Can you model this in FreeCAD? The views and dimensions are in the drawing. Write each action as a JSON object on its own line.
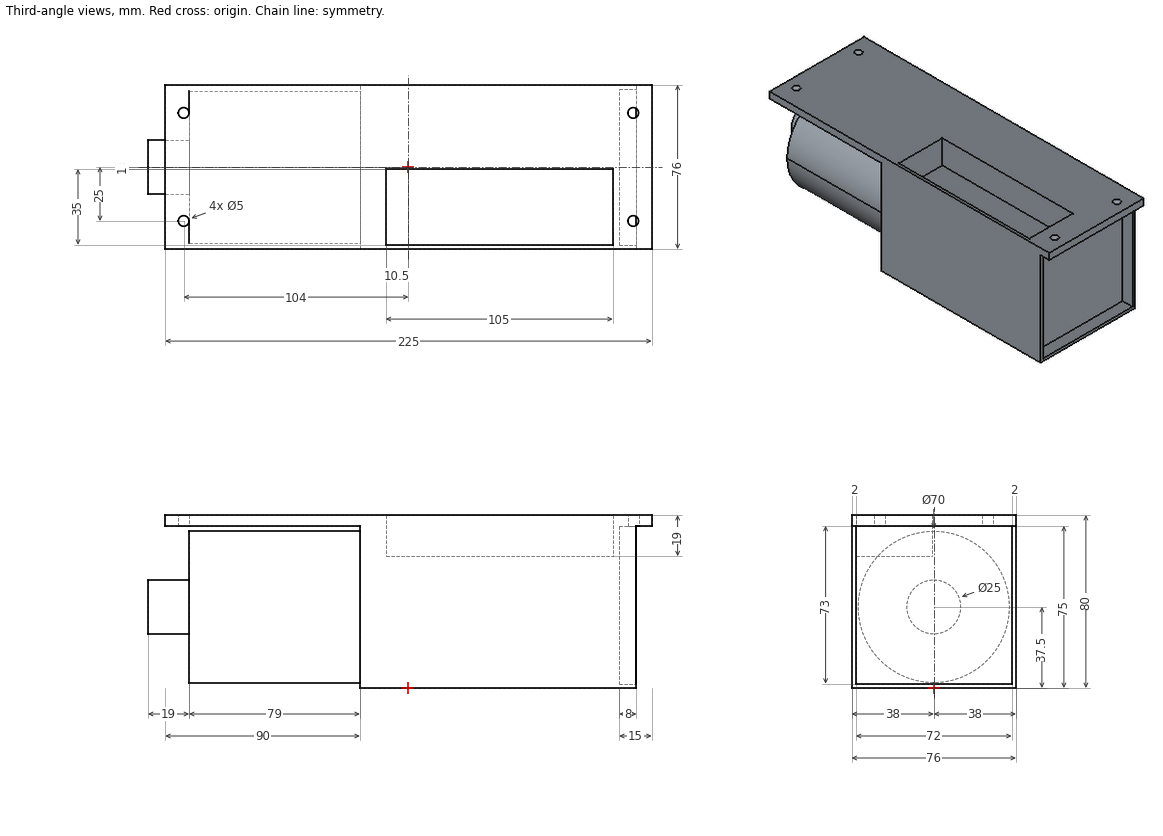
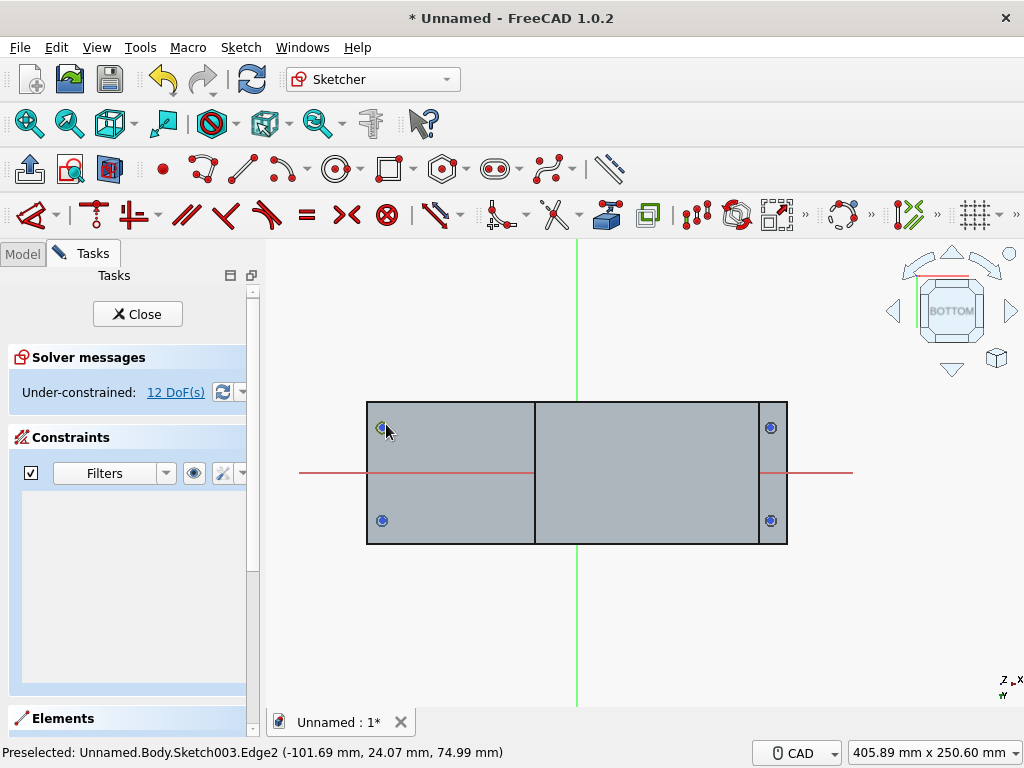
{"action": "scroll", "coordinate": [775, 424], "scroll_direction": "up", "scroll_amount": 5}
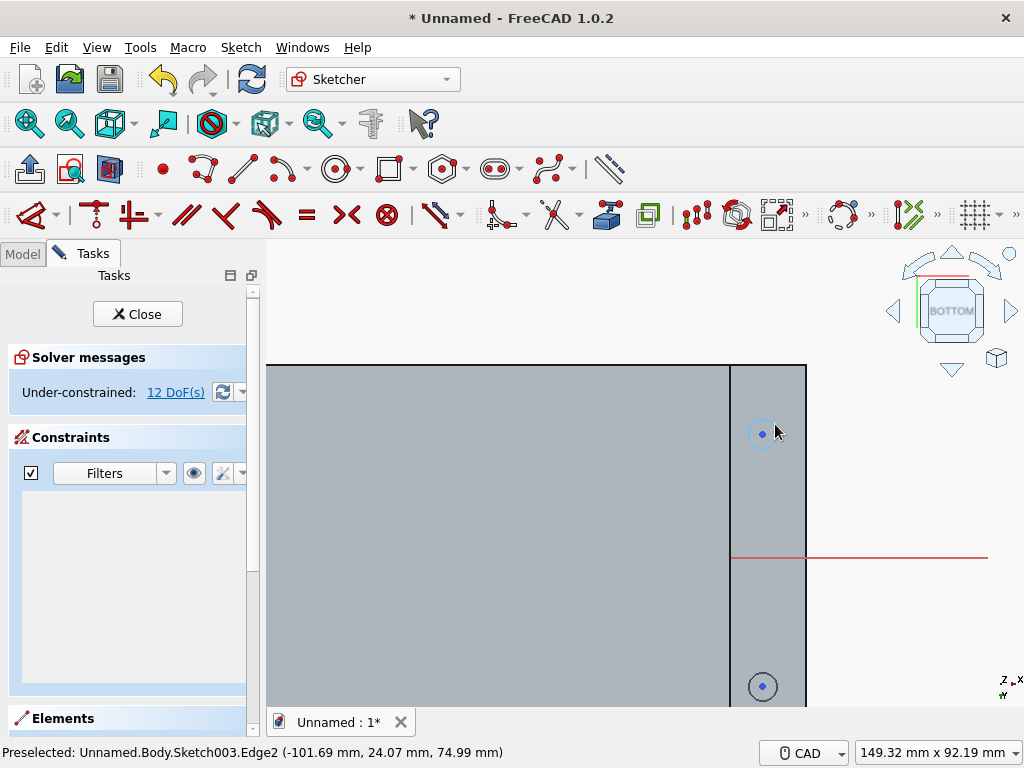
{"action": "left_click", "coordinate": [773, 424]}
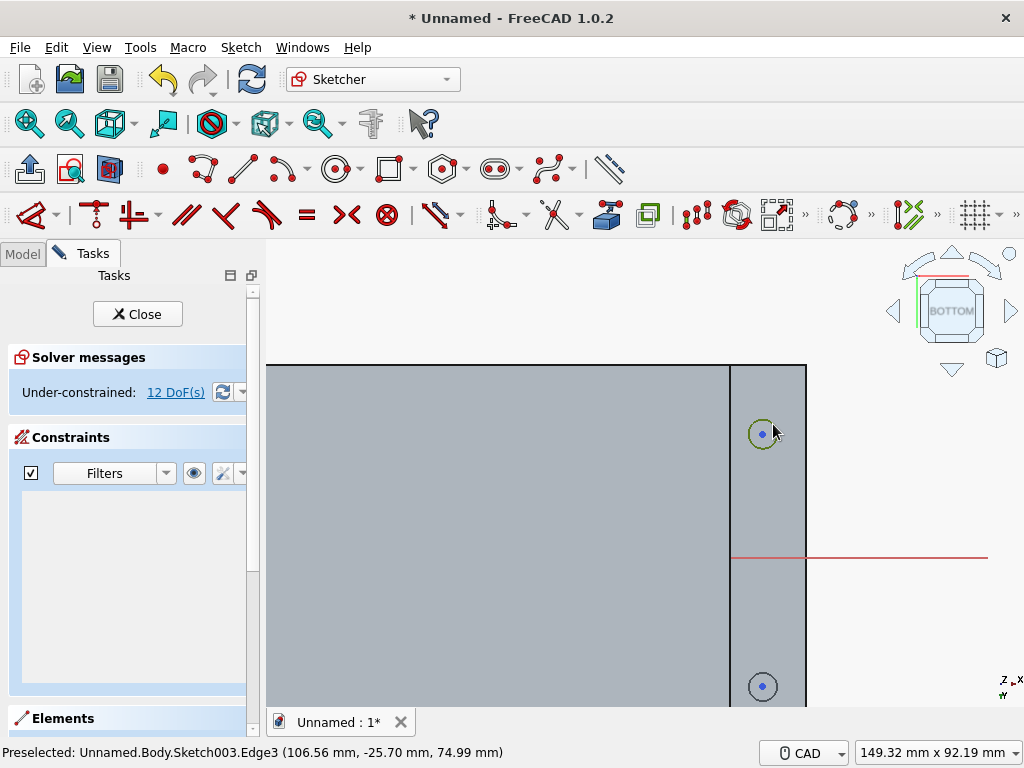
{"action": "left_click", "coordinate": [773, 677]}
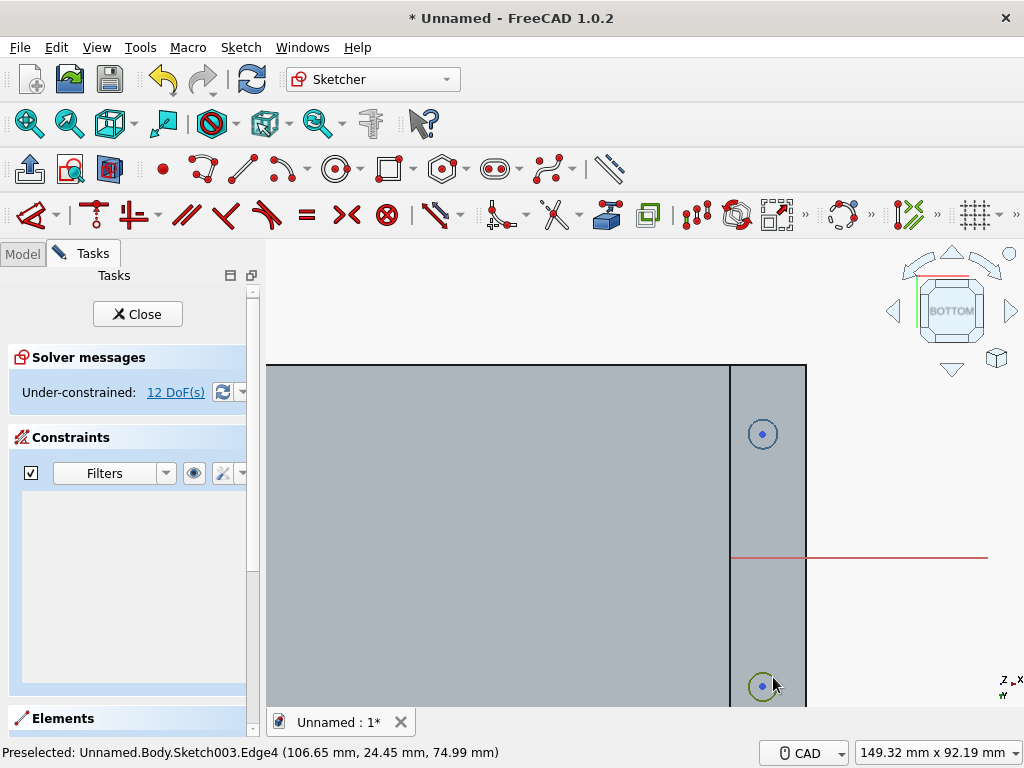
{"action": "left_click", "coordinate": [308, 216]}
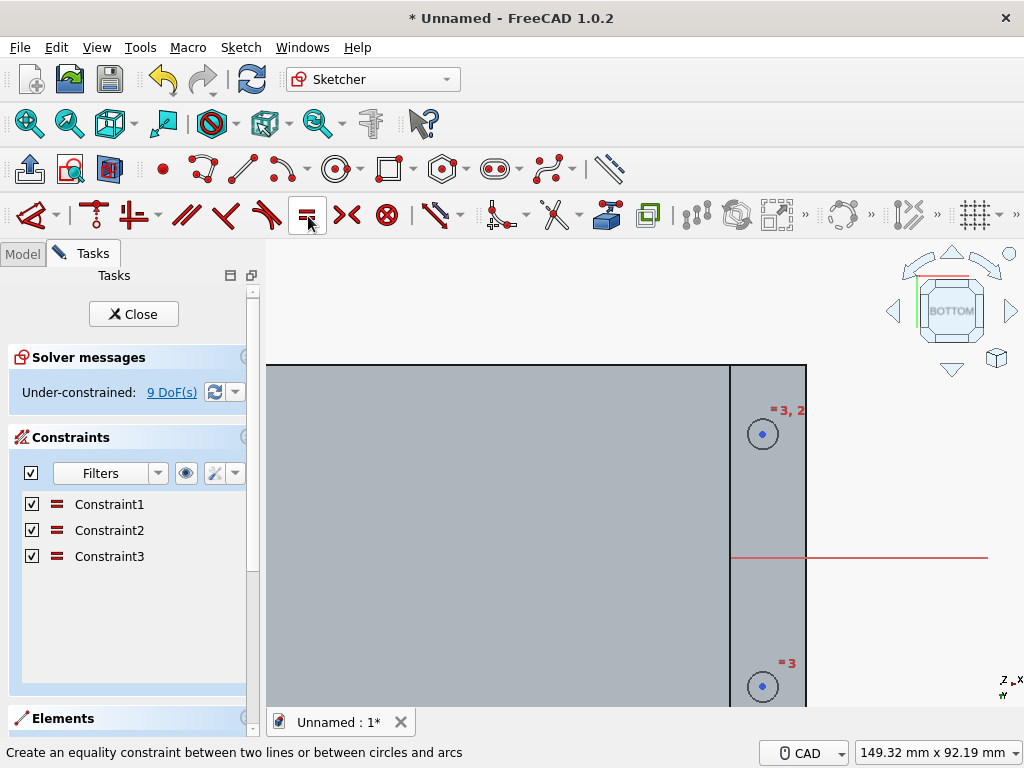
{"action": "scroll", "coordinate": [775, 424], "scroll_direction": "down", "scroll_amount": 5}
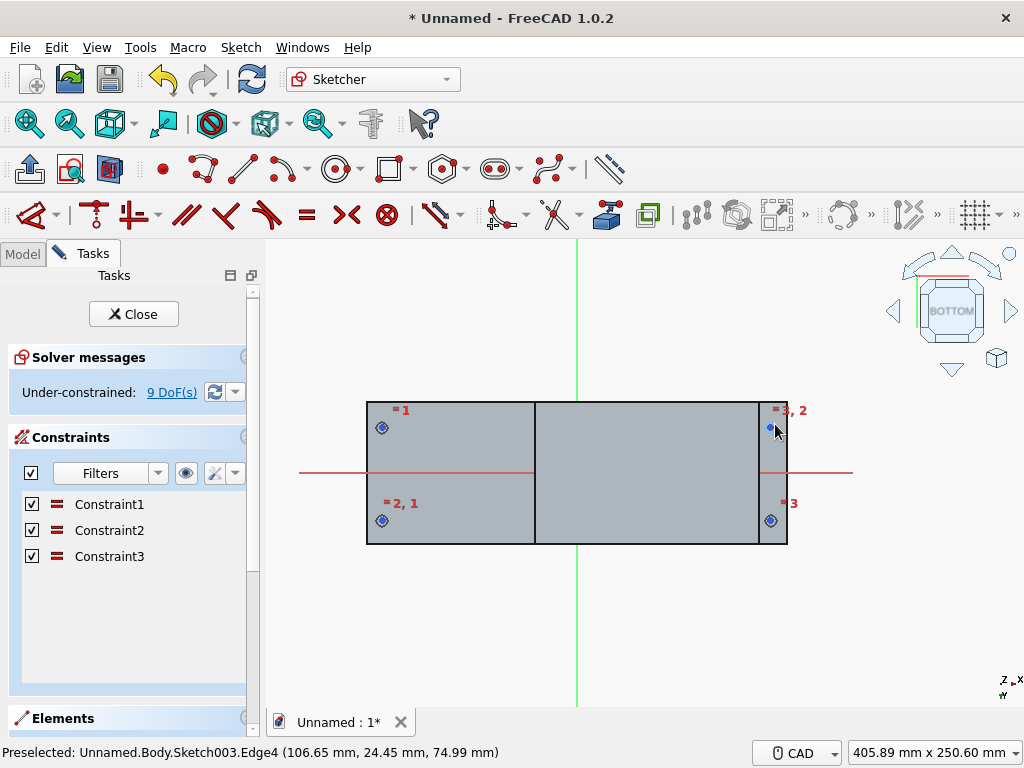
{"action": "left_click", "coordinate": [382, 428]}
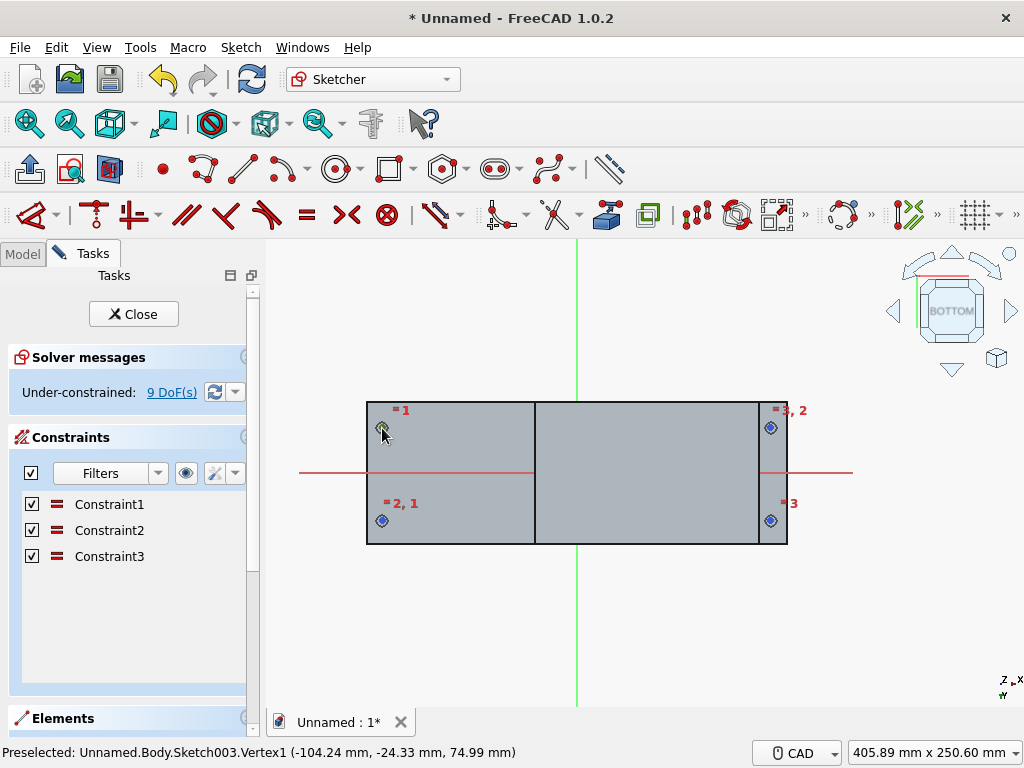
{"action": "left_click", "coordinate": [382, 521]}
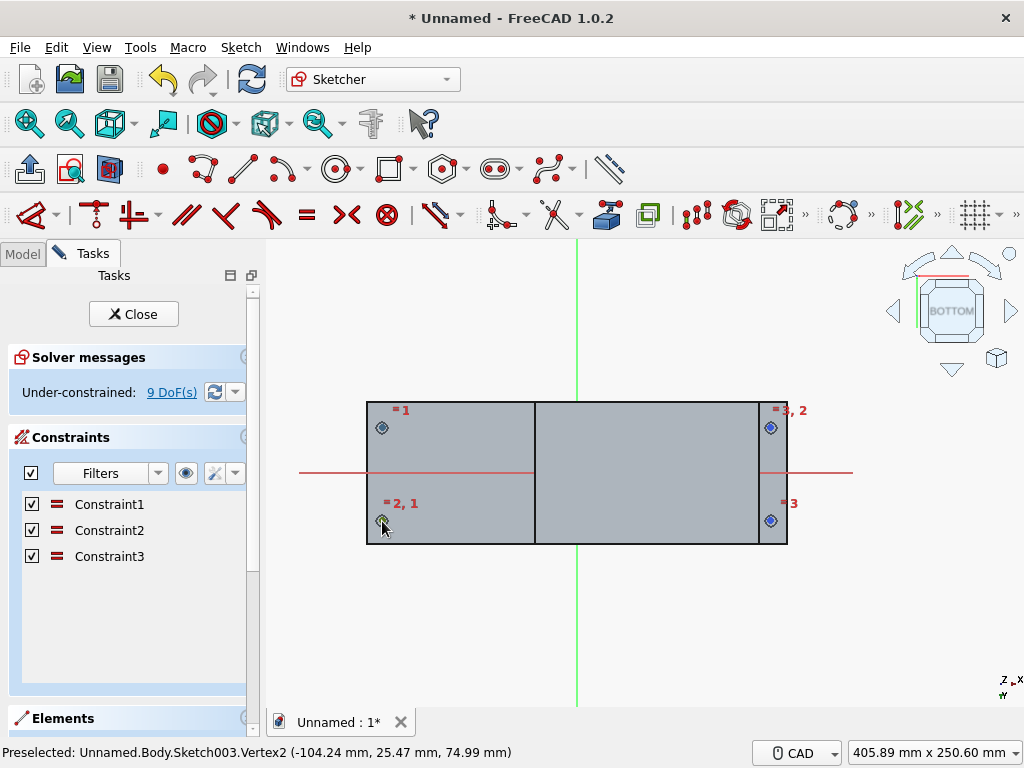
{"action": "left_click", "coordinate": [334, 473]}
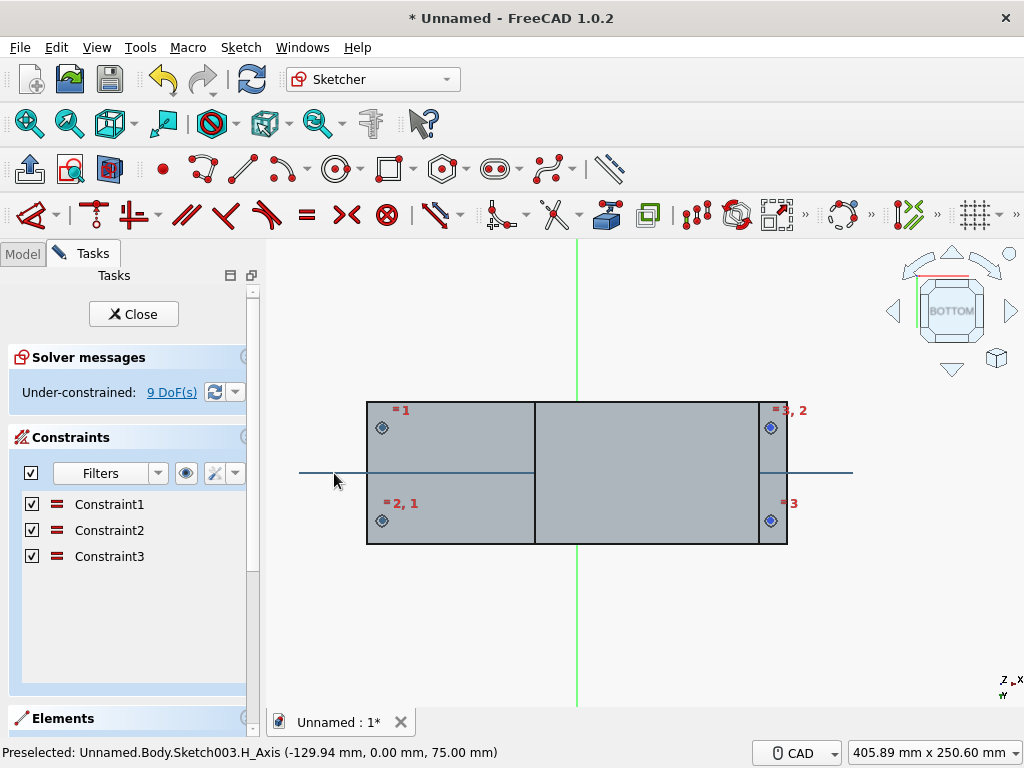
{"action": "key", "text": "s"}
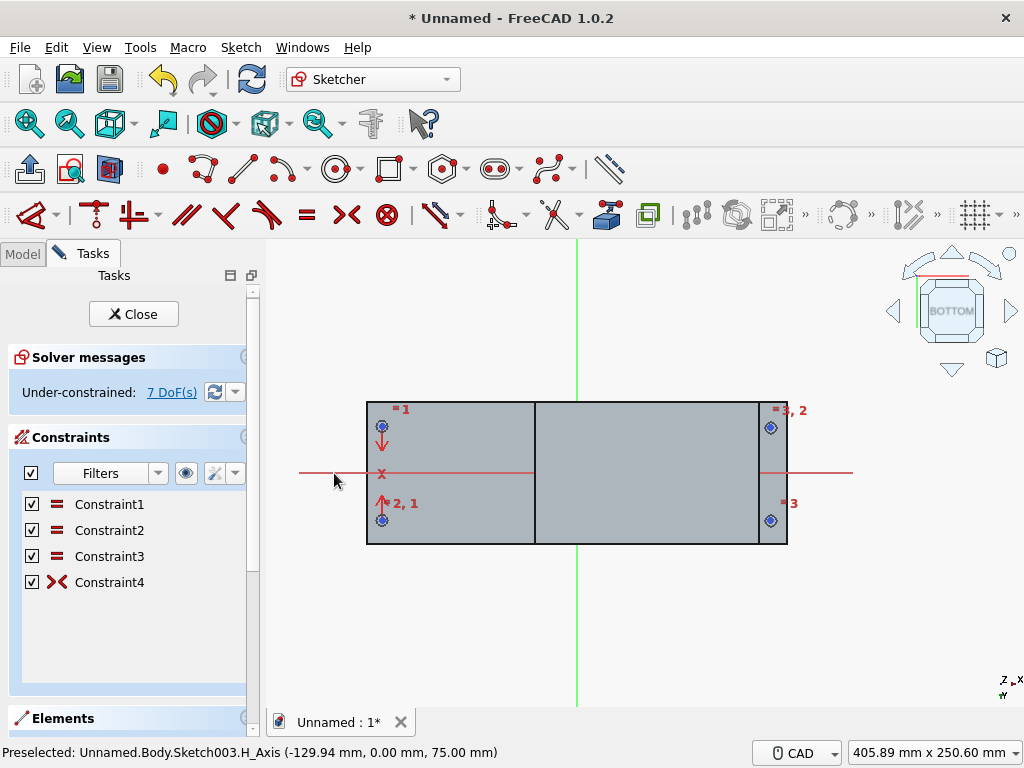
{"action": "left_click", "coordinate": [382, 426]}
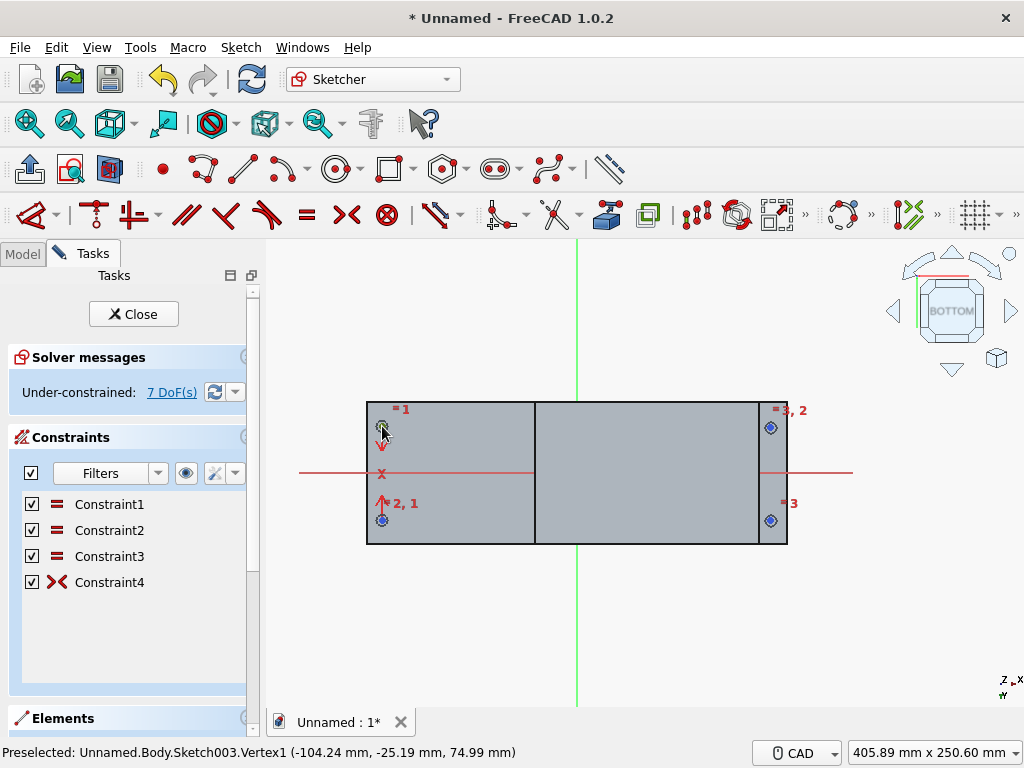
{"action": "left_click", "coordinate": [771, 428]}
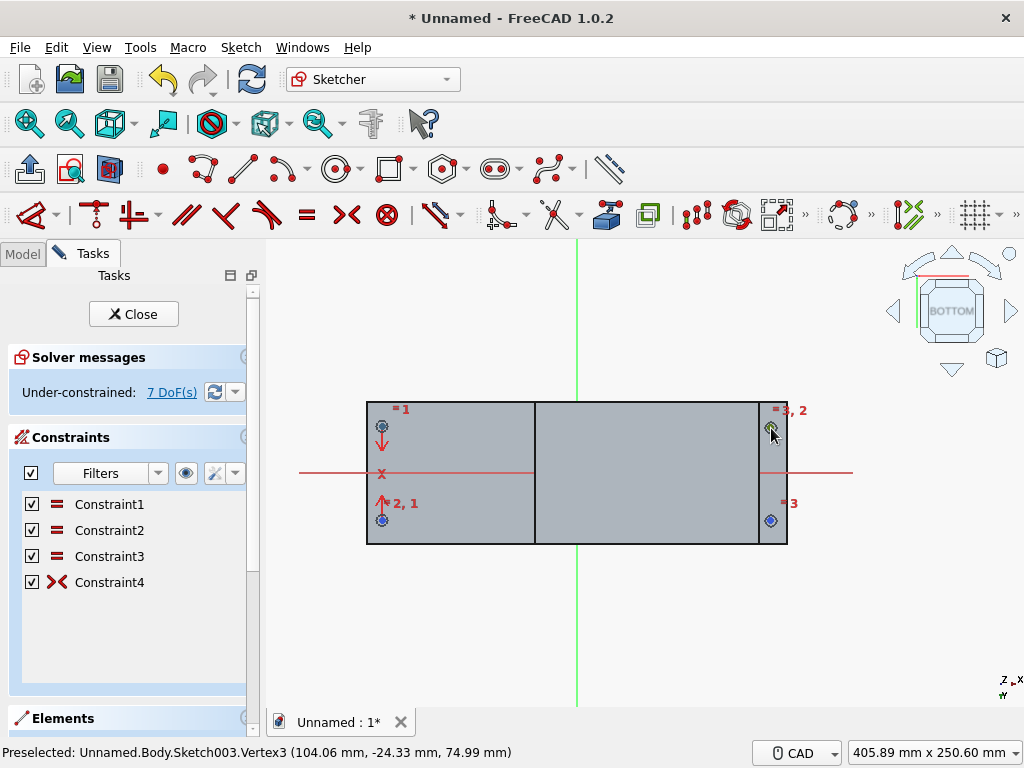
{"action": "left_click", "coordinate": [577, 650]}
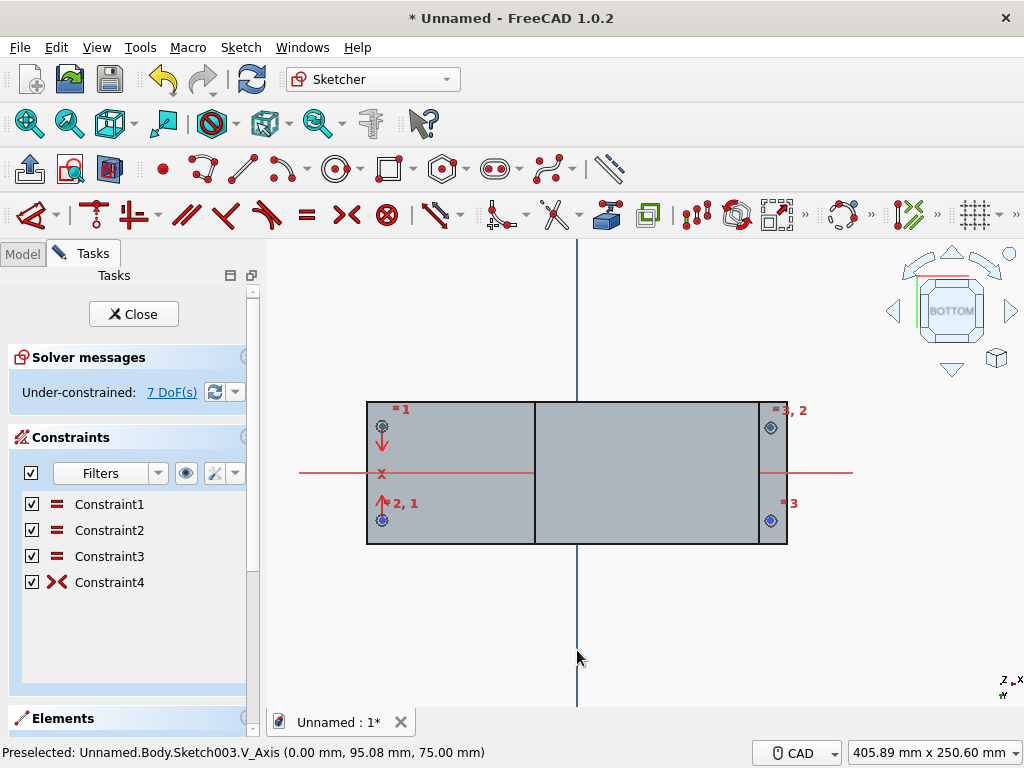
{"action": "left_click", "coordinate": [348, 216]}